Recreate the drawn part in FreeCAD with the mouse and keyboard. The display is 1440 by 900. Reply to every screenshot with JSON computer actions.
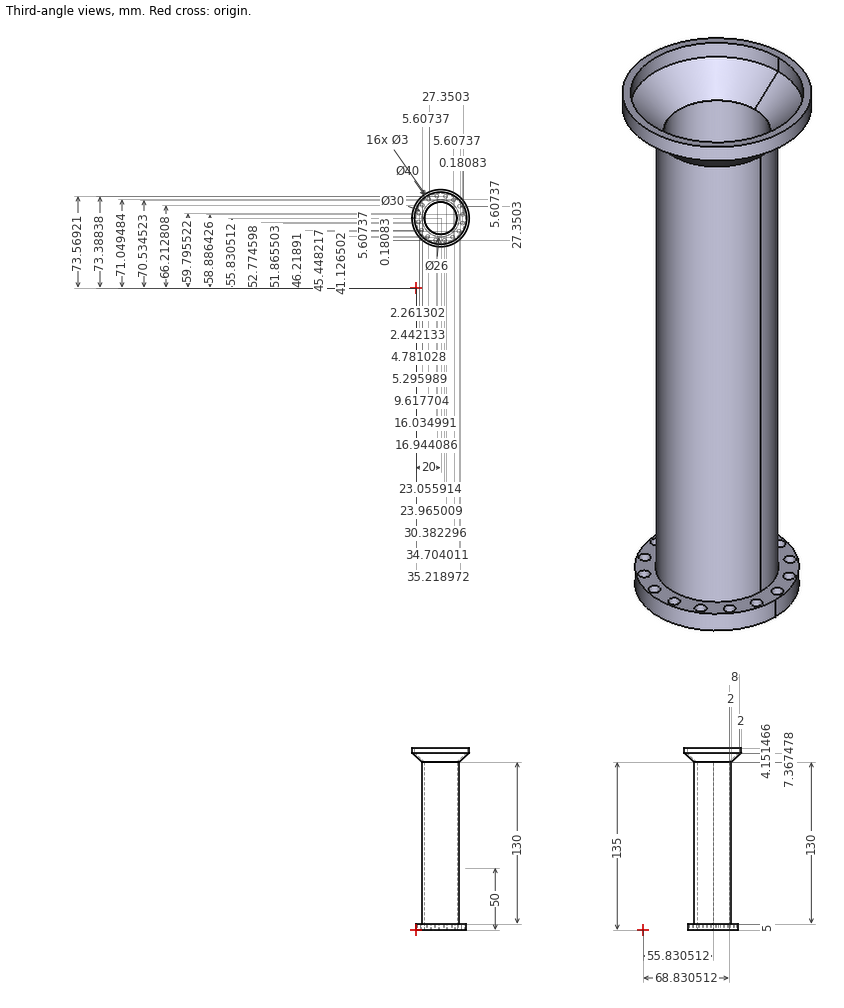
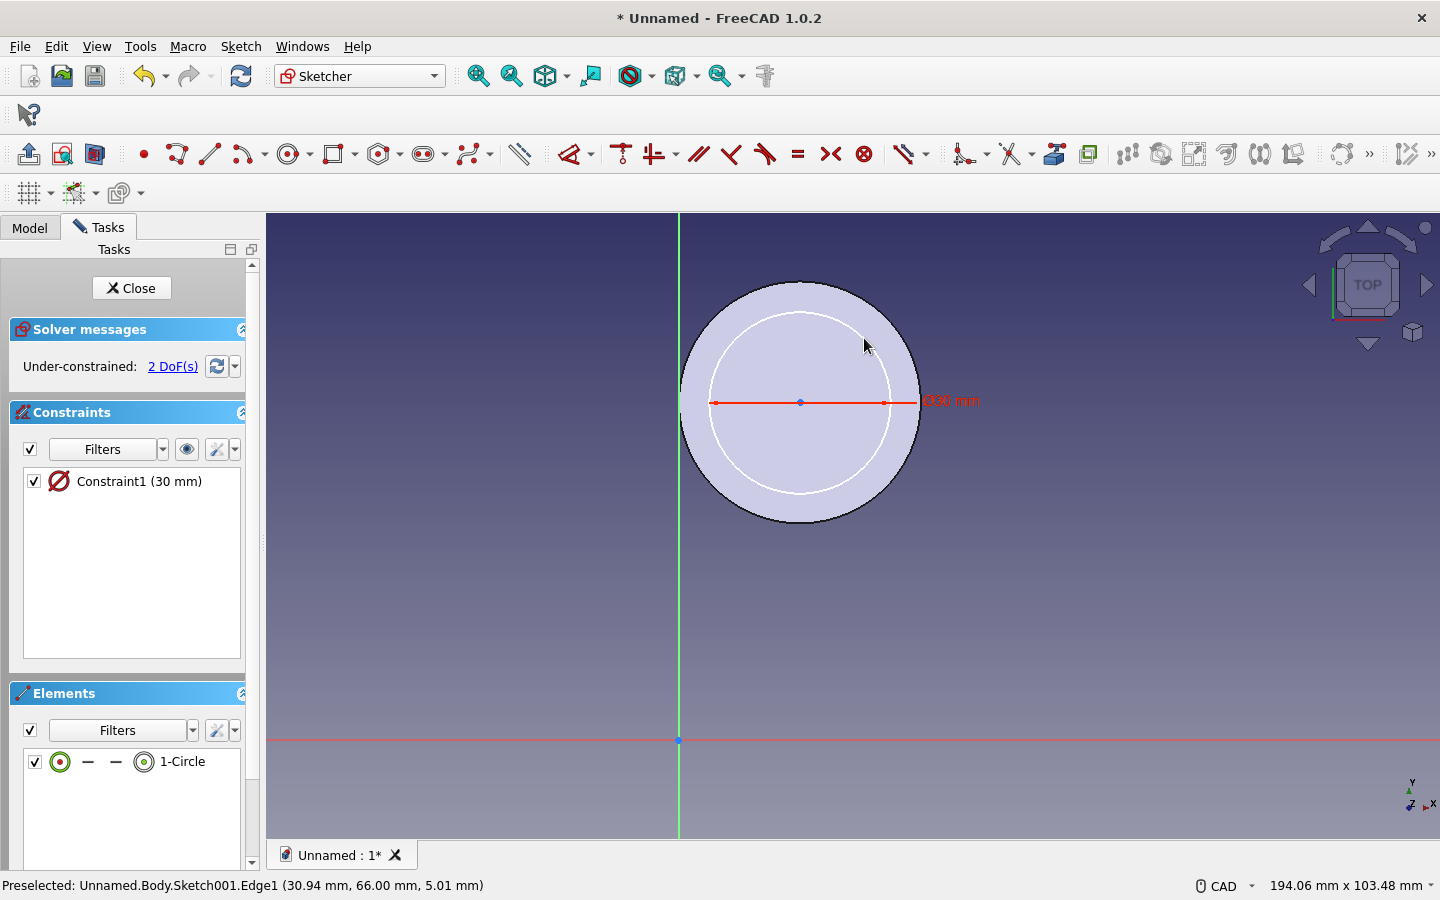
{"action": "left_click", "coordinate": [568, 154]}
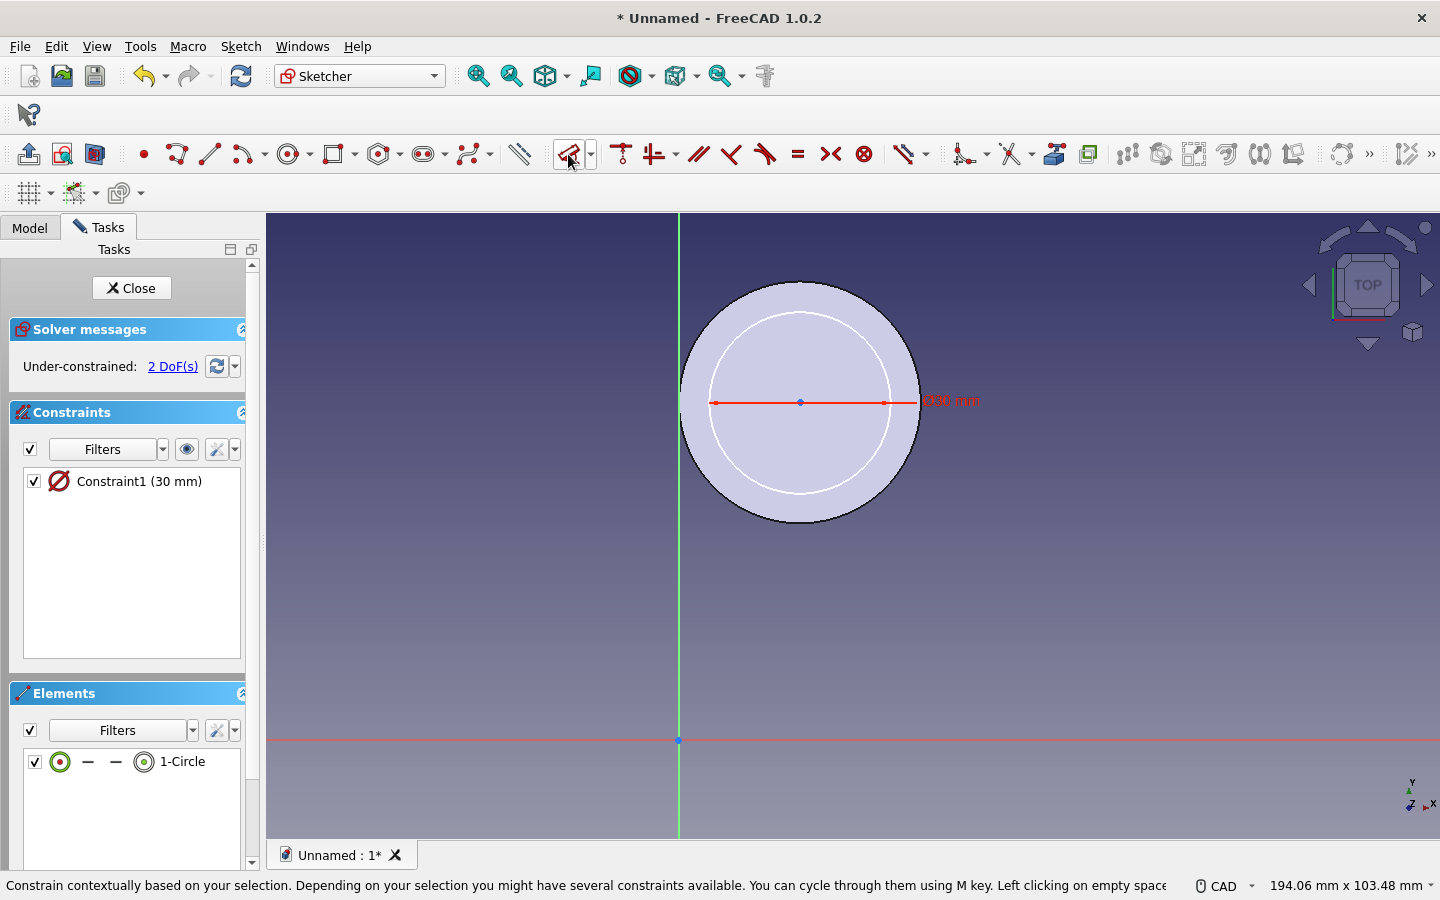
{"action": "left_click", "coordinate": [800, 403]}
{"action": "left_click", "coordinate": [739, 774]}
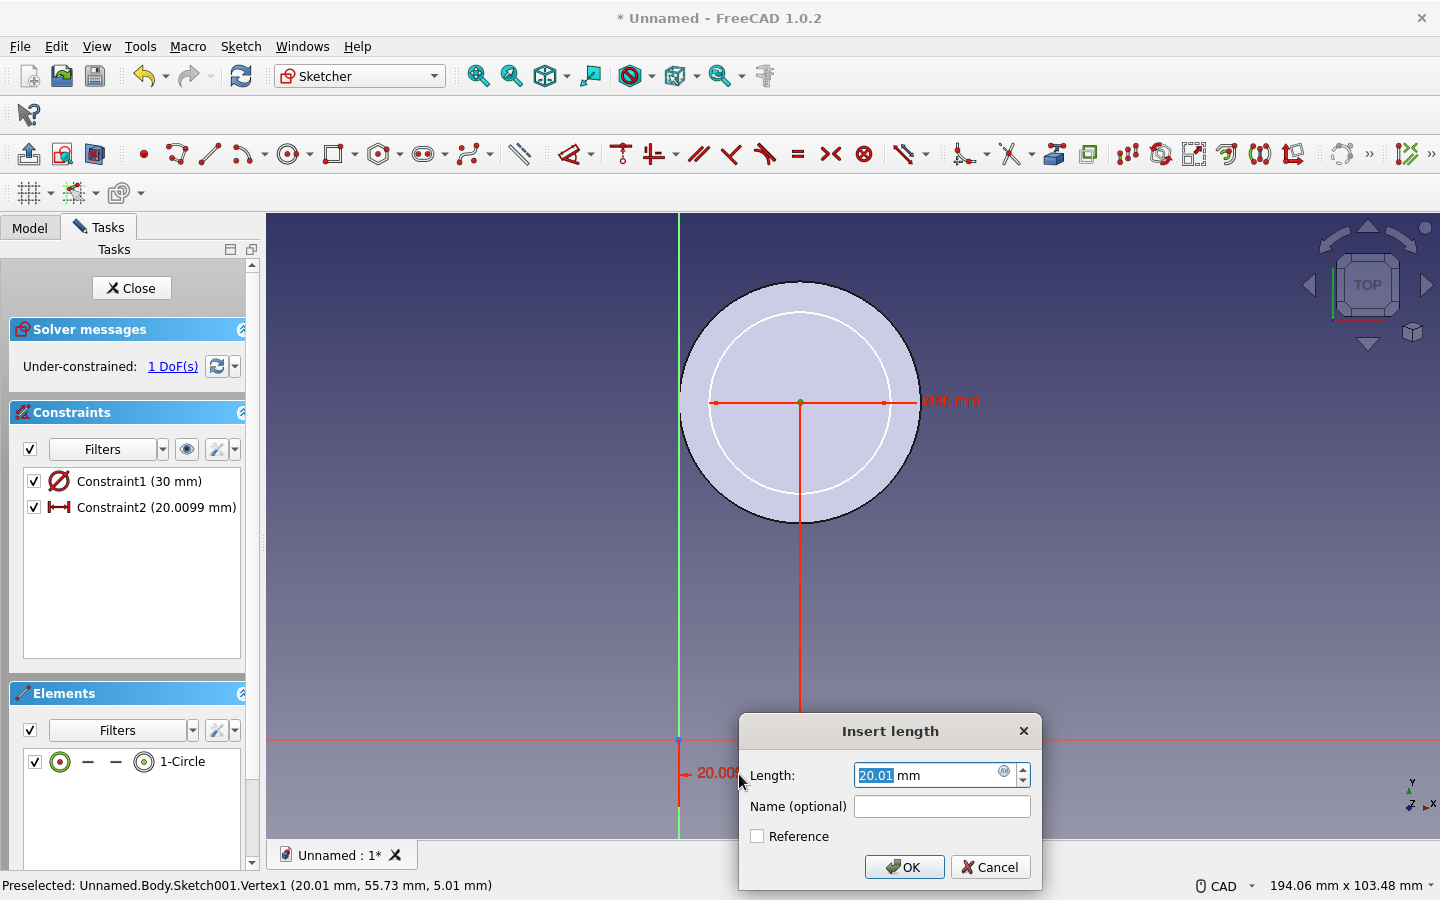
{"action": "type", "text": "20"}
{"action": "key", "text": "Return"}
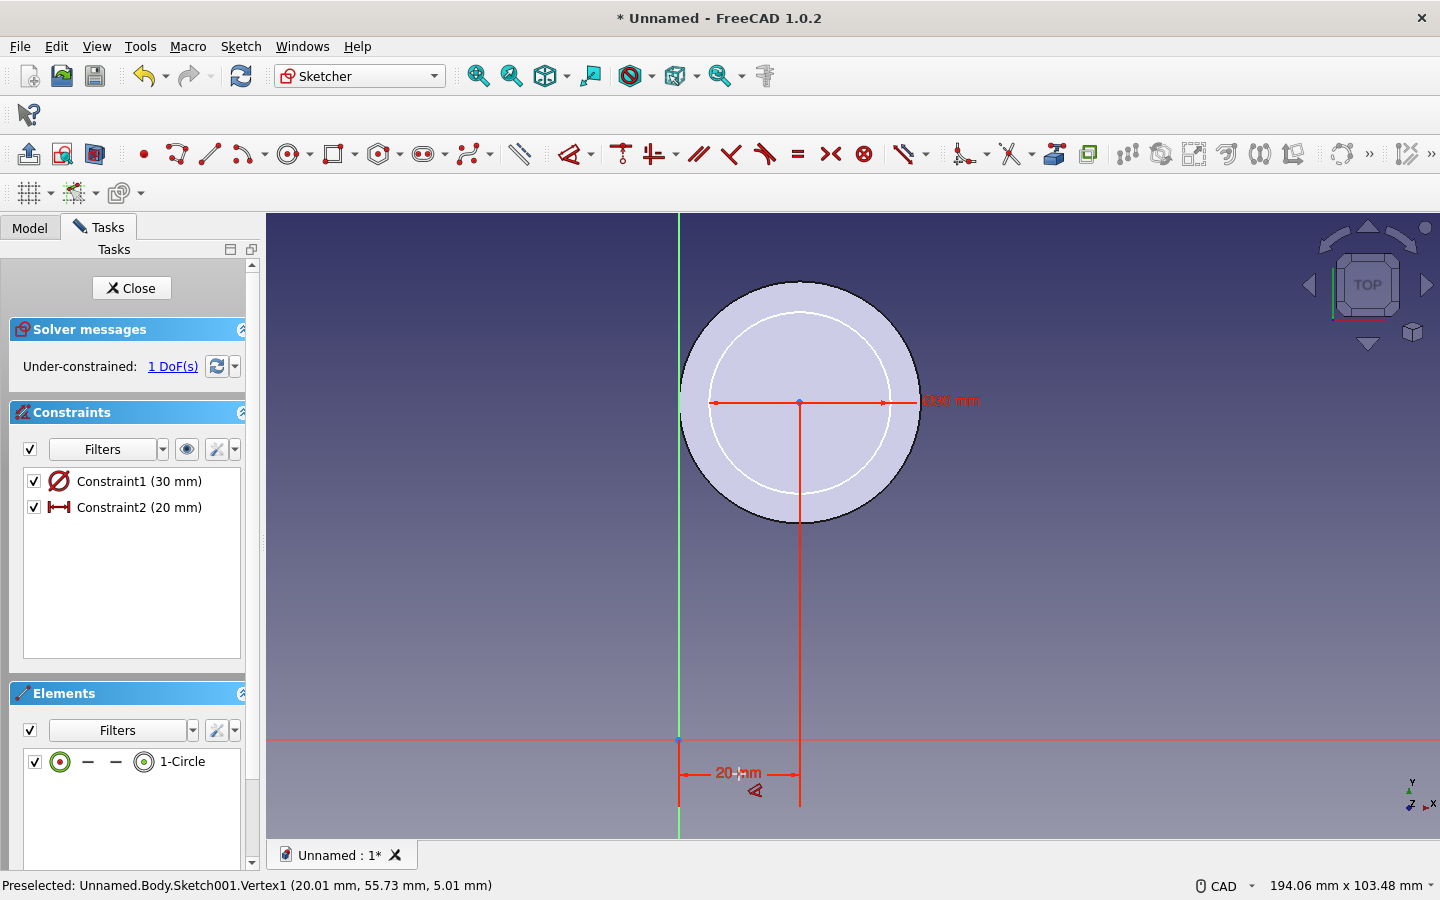
{"action": "left_click", "coordinate": [800, 403]}
{"action": "left_click", "coordinate": [645, 572]}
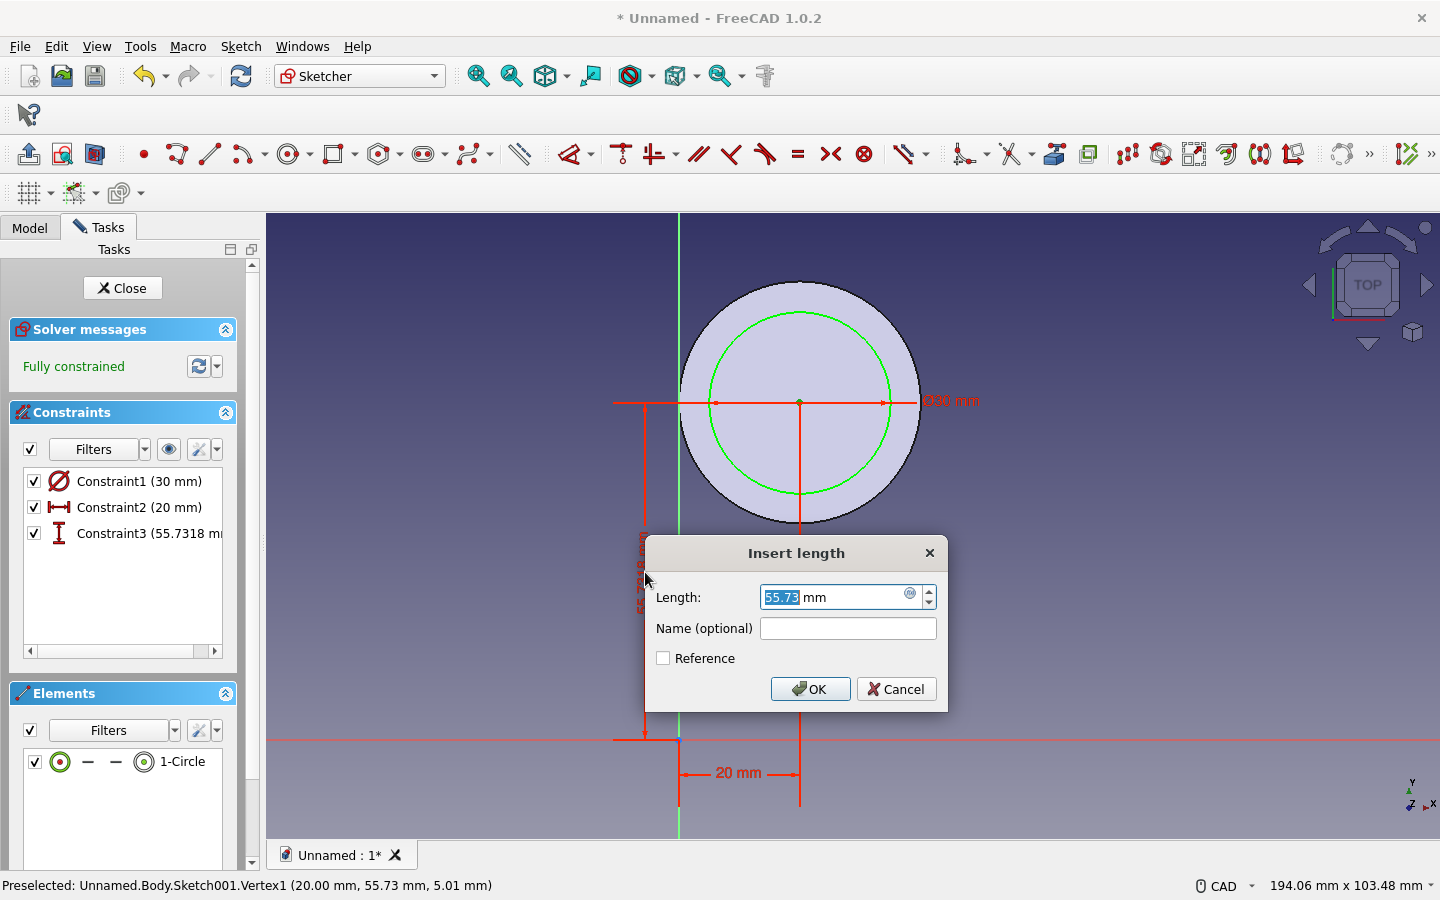
{"action": "type", "text": "55.830512"}
{"action": "key", "text": "Return"}
{"action": "key", "text": "Escape"}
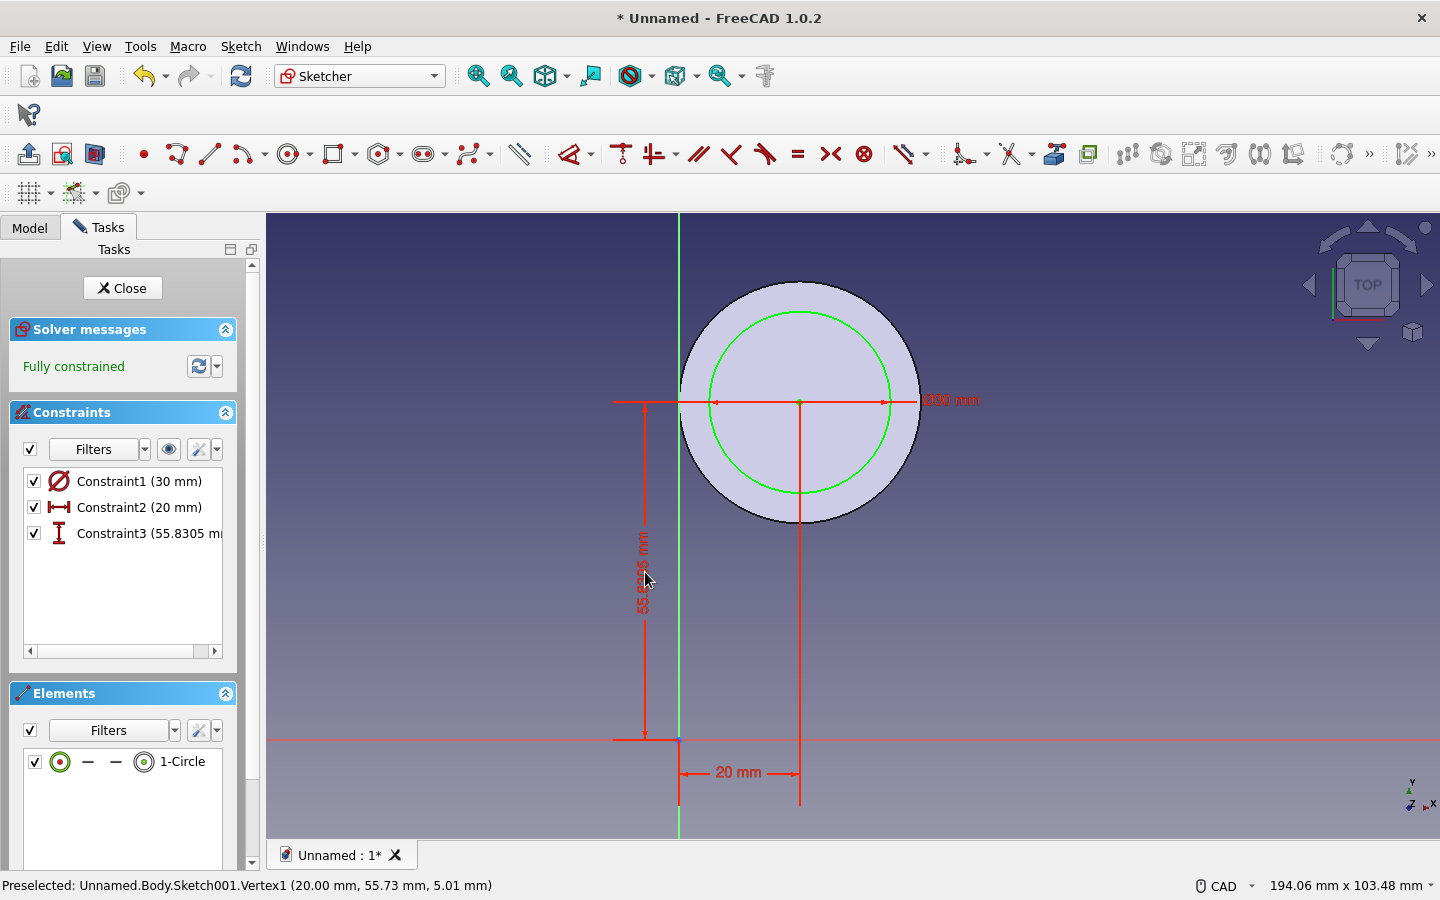
{"action": "left_click", "coordinate": [123, 288]}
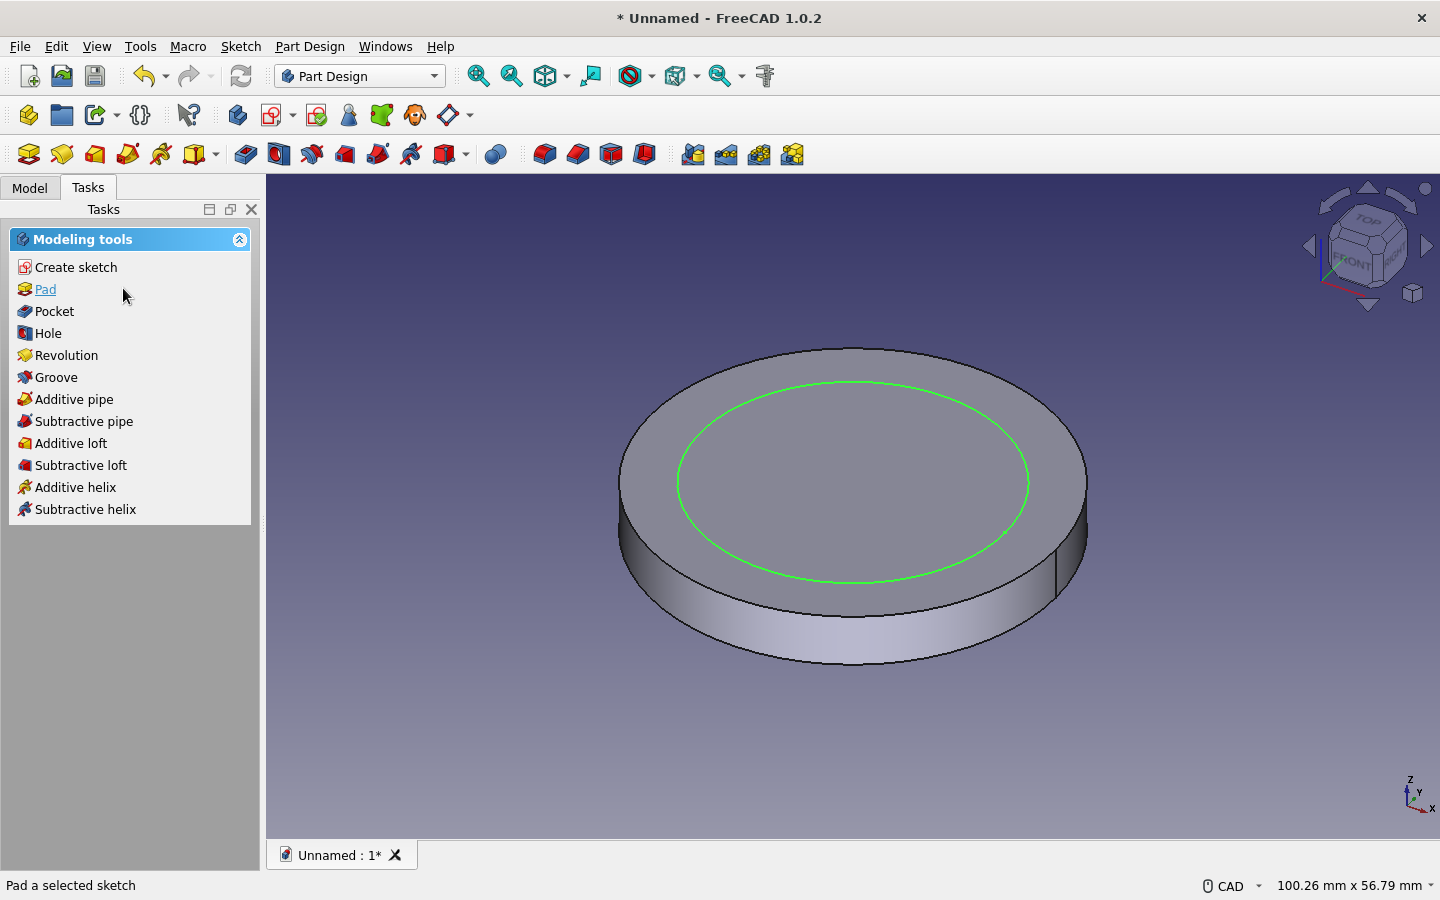
{"action": "left_click", "coordinate": [29, 154]}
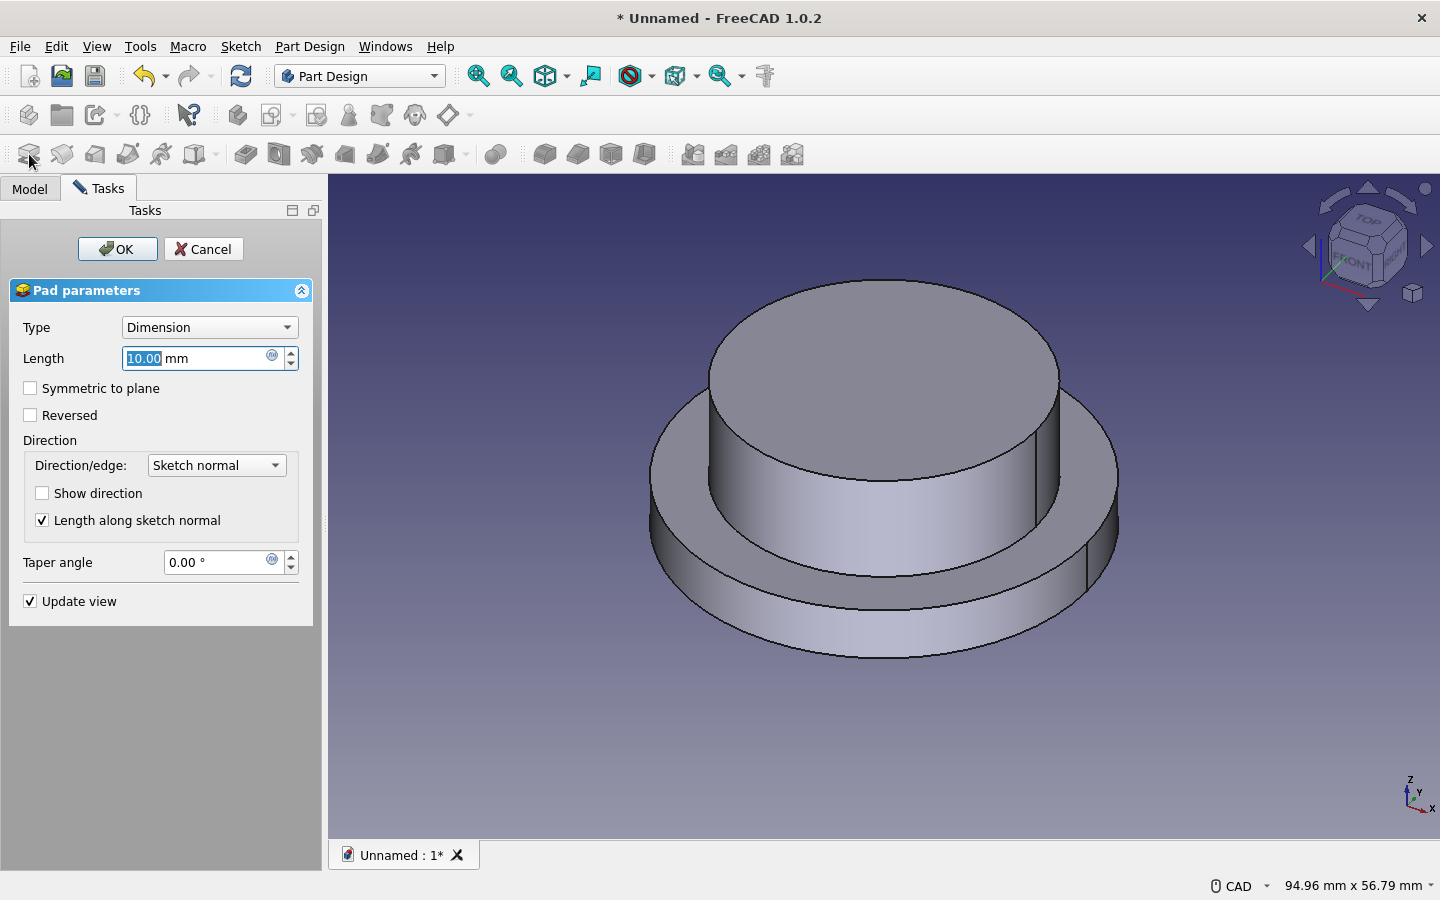
{"action": "type", "text": "130"}
{"action": "key", "text": "Tab"}